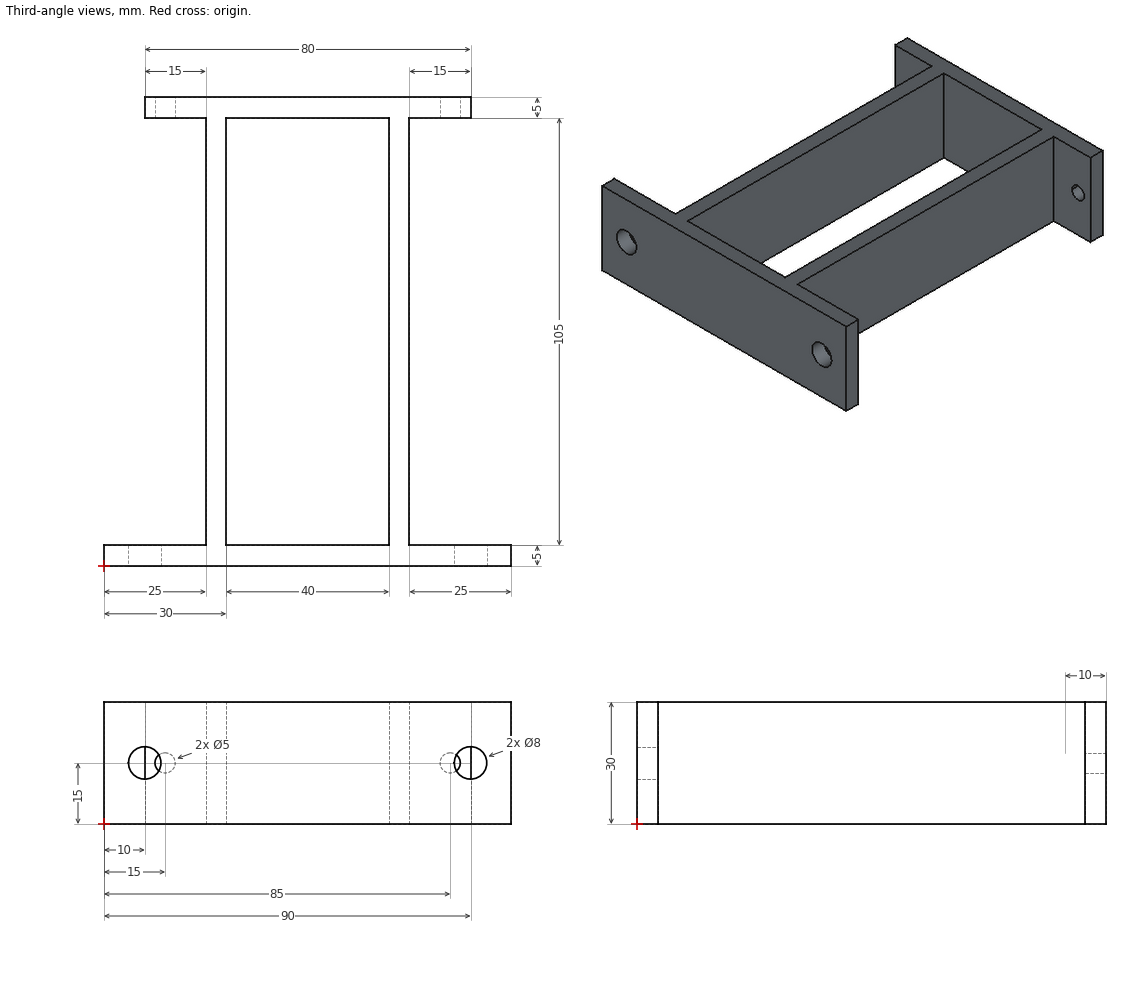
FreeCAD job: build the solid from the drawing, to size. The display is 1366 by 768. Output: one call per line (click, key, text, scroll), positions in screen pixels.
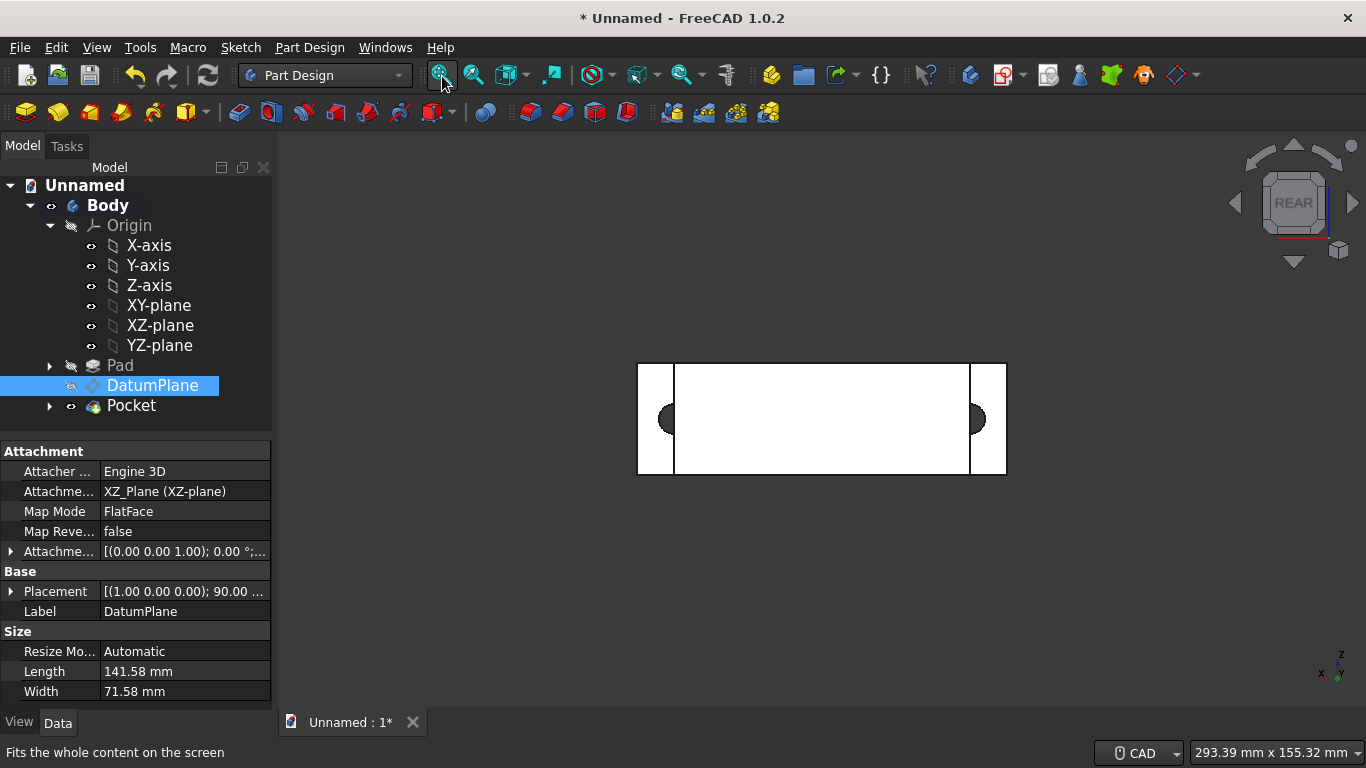
click(442, 76)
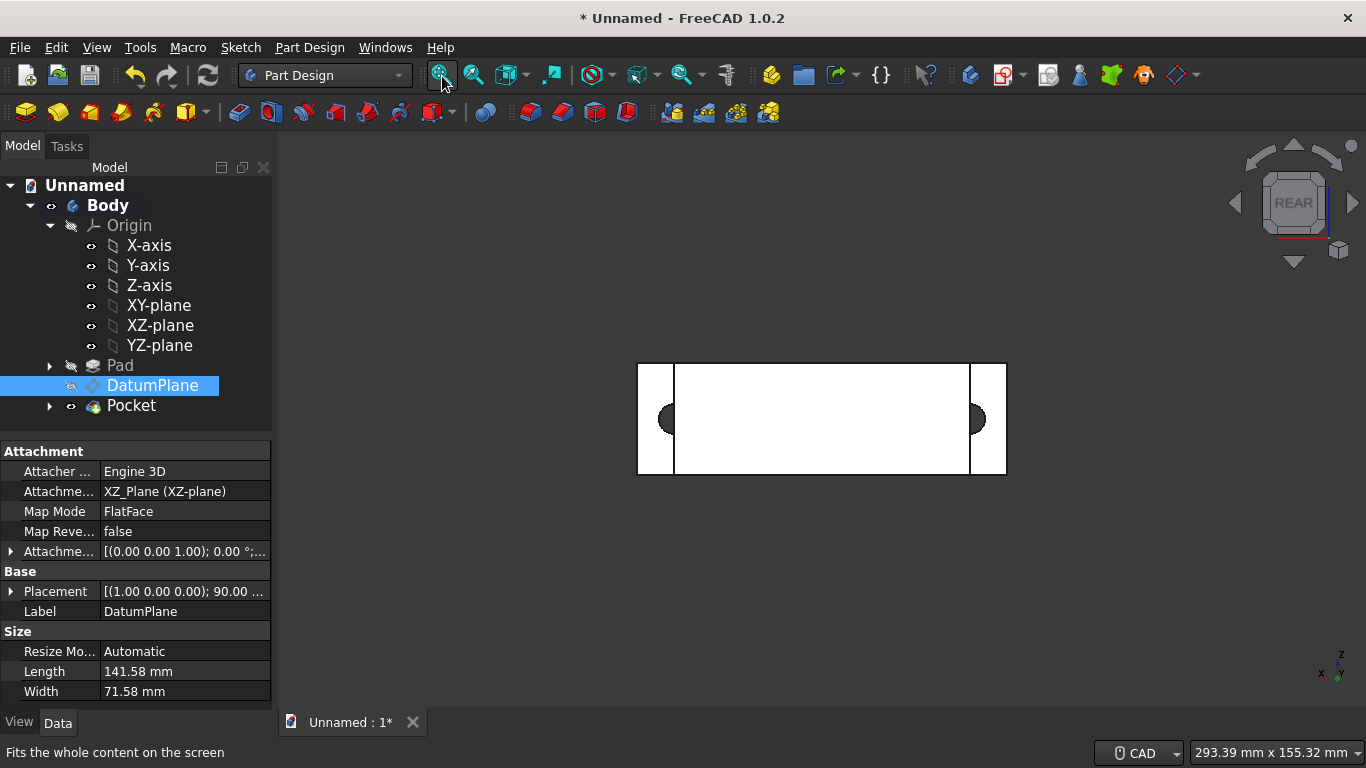
click(737, 418)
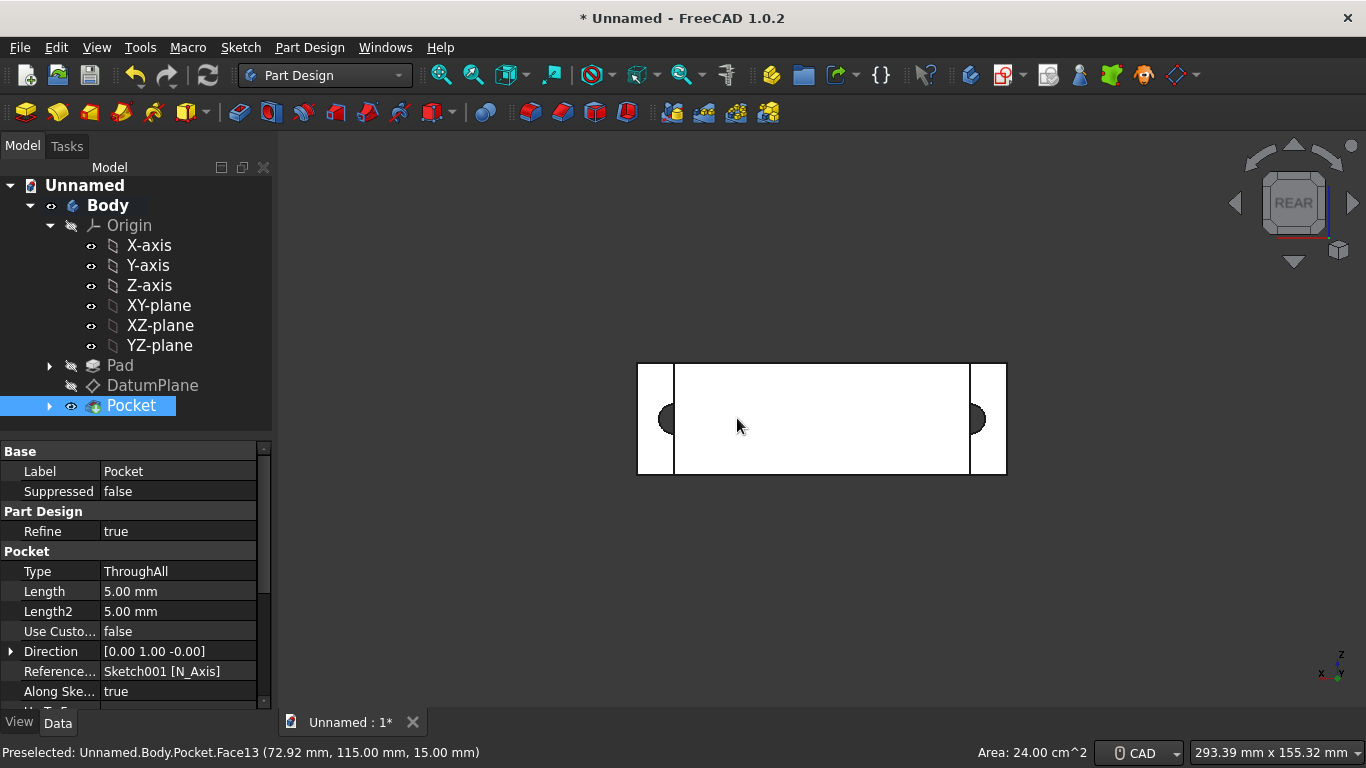
click(1004, 76)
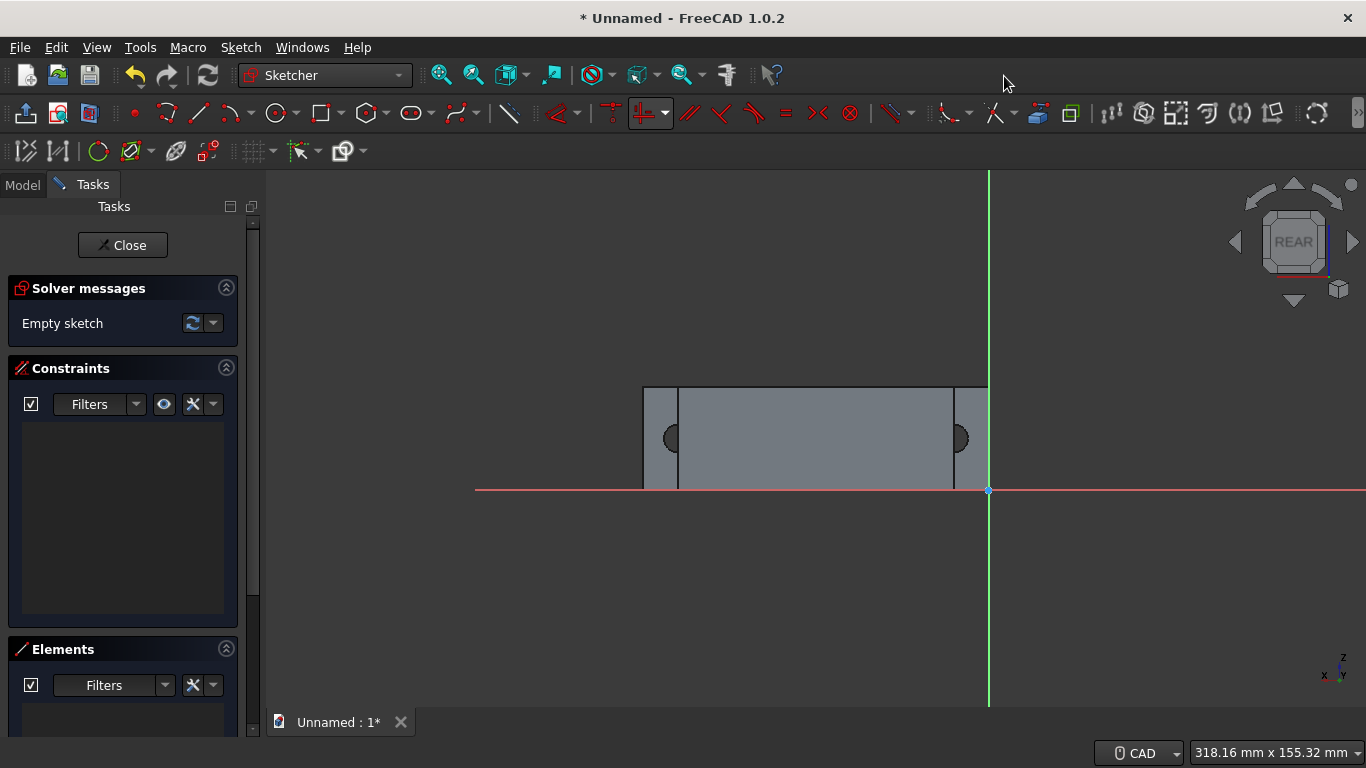
scroll(911, 478, up, 4)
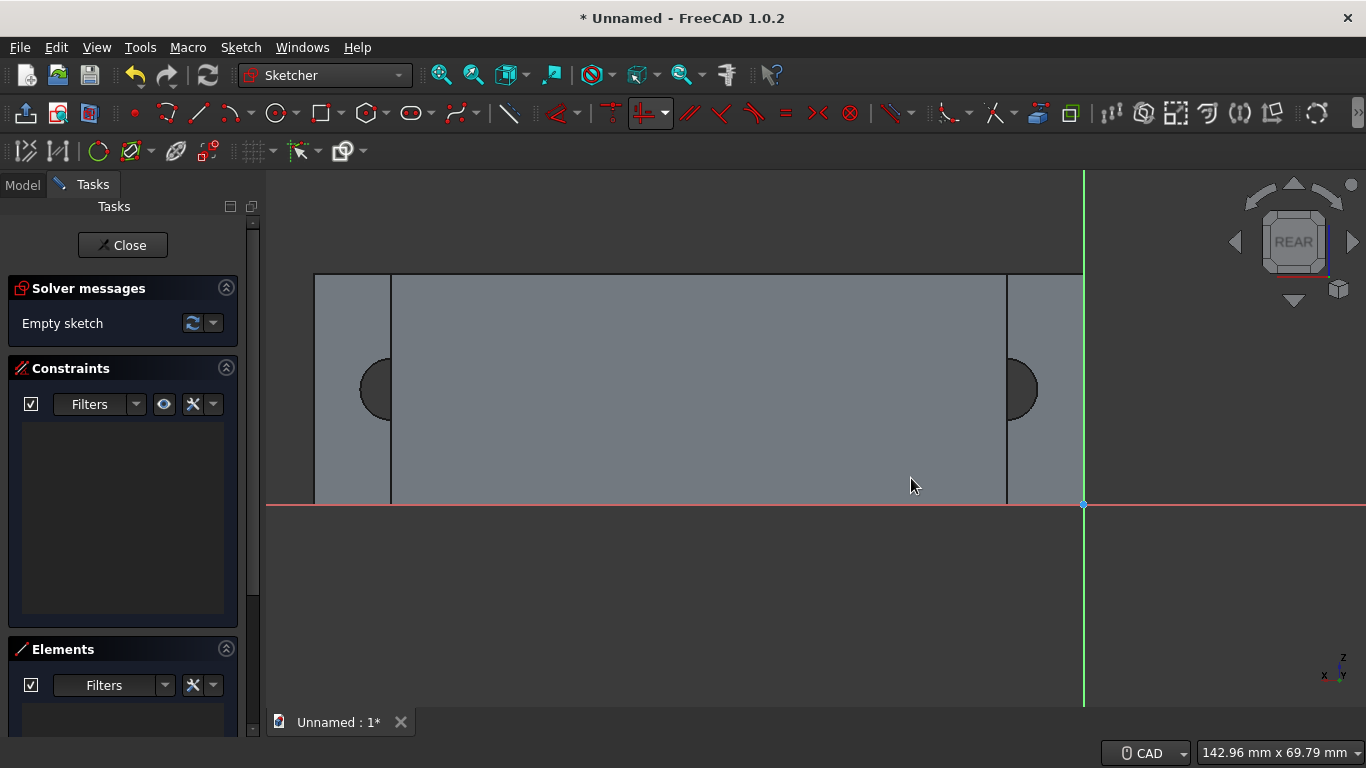
click(276, 114)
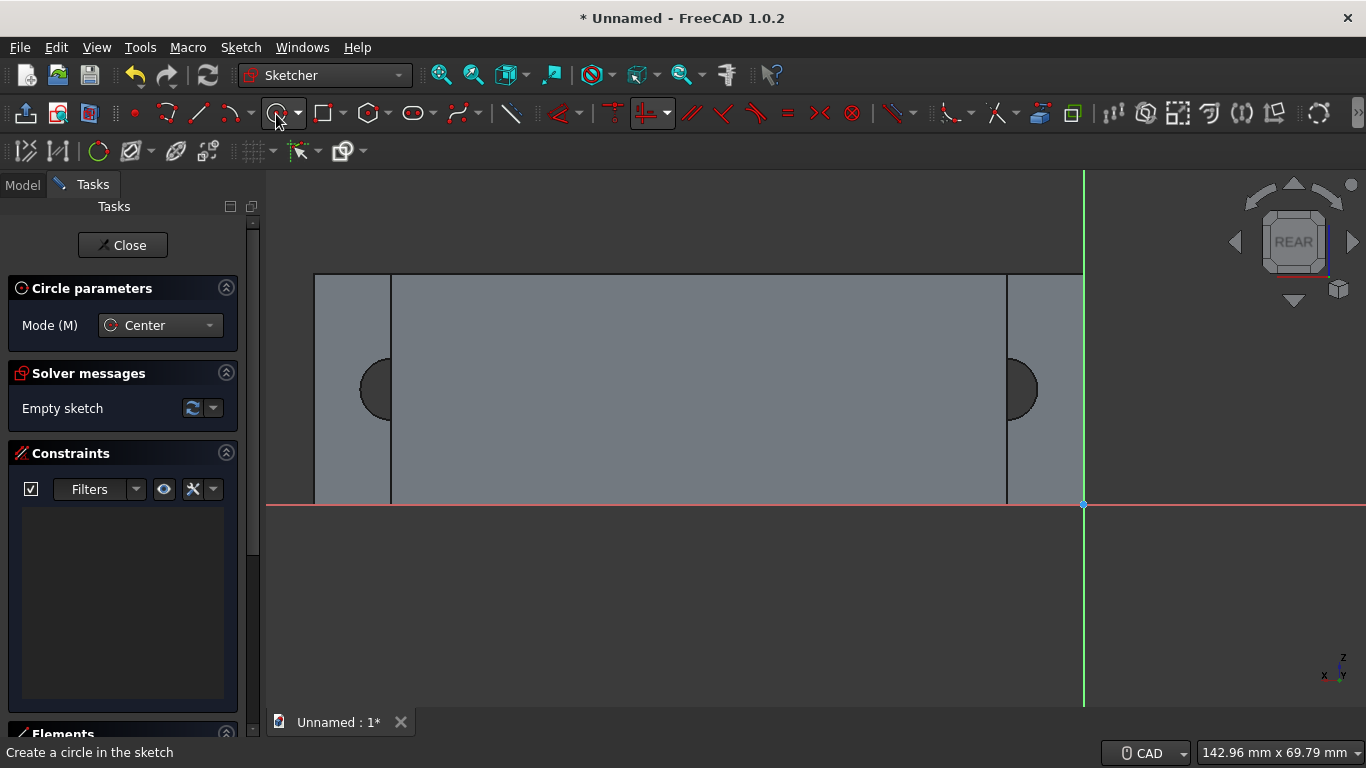
click(968, 389)
click(982, 376)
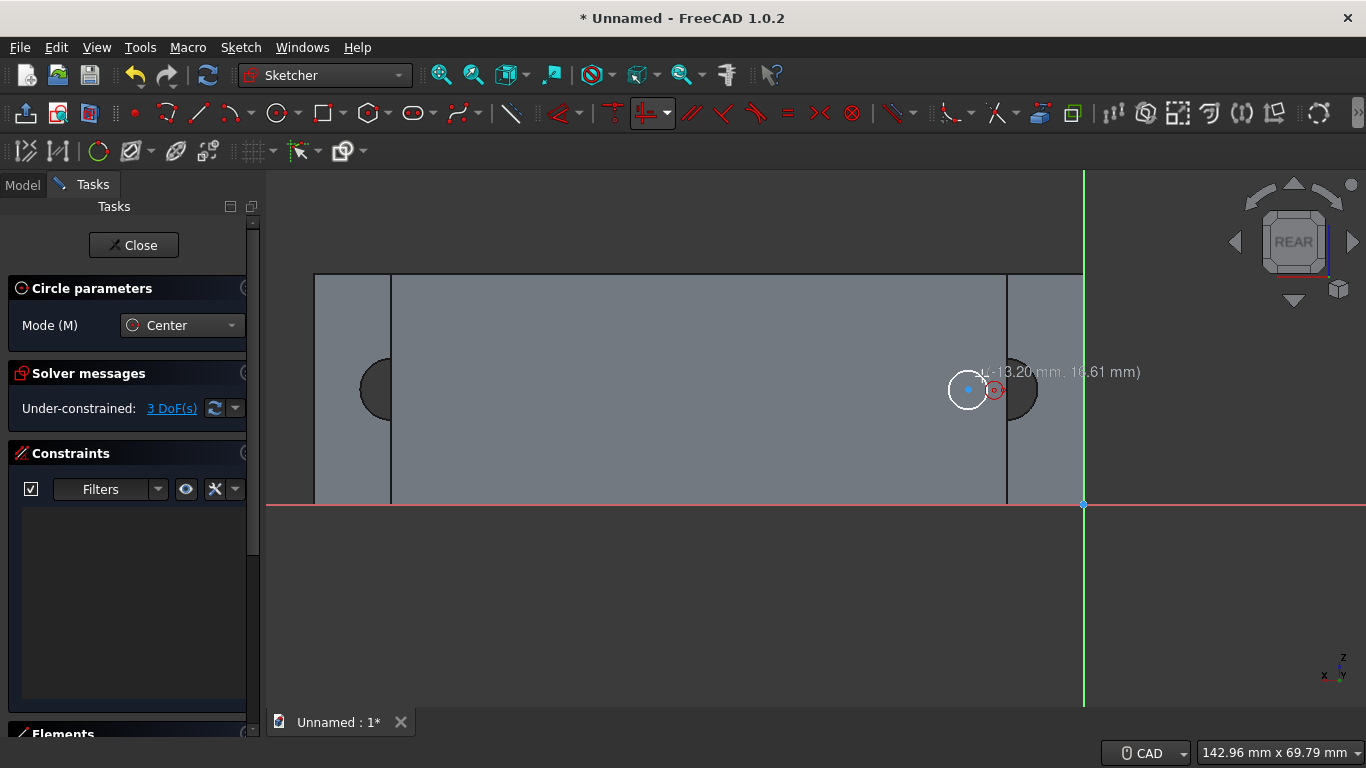
click(430, 389)
click(443, 376)
key(Escape)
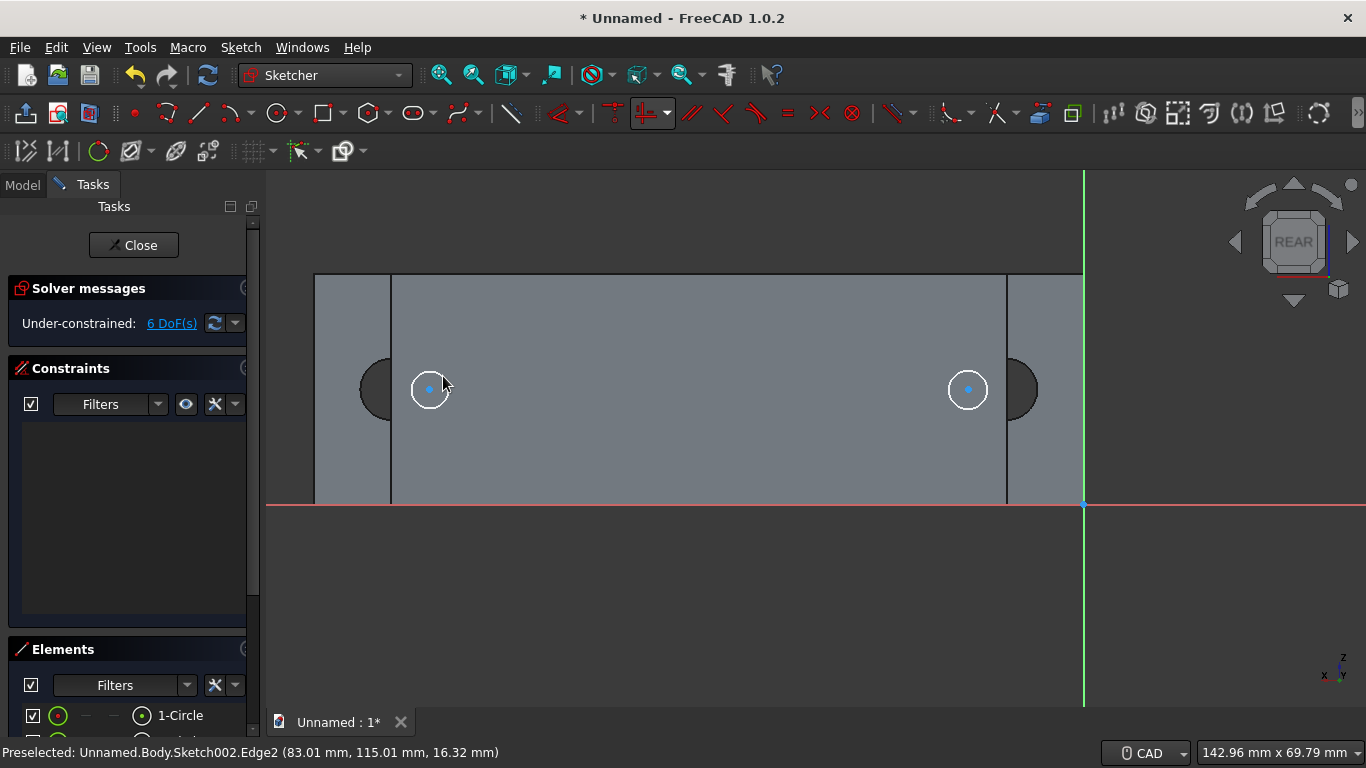
click(981, 376)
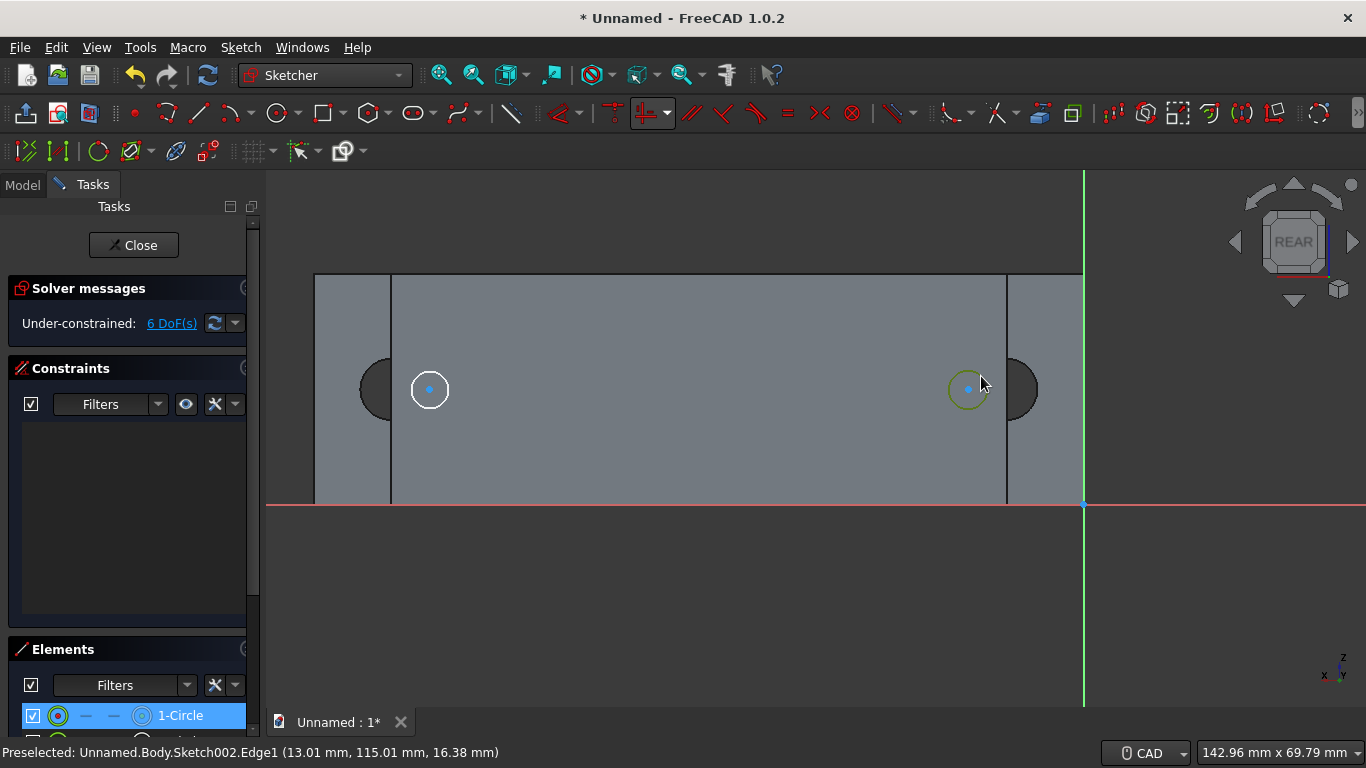
click(443, 377)